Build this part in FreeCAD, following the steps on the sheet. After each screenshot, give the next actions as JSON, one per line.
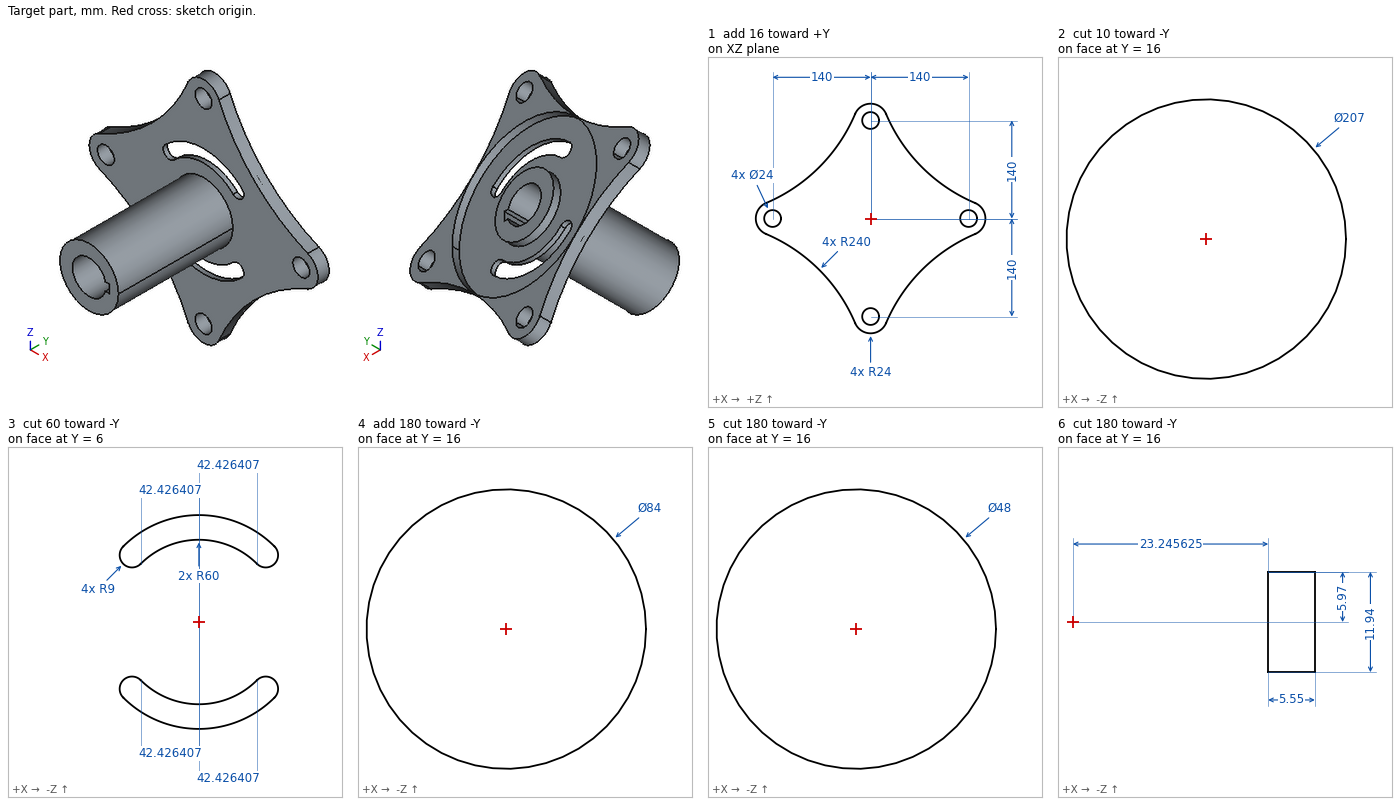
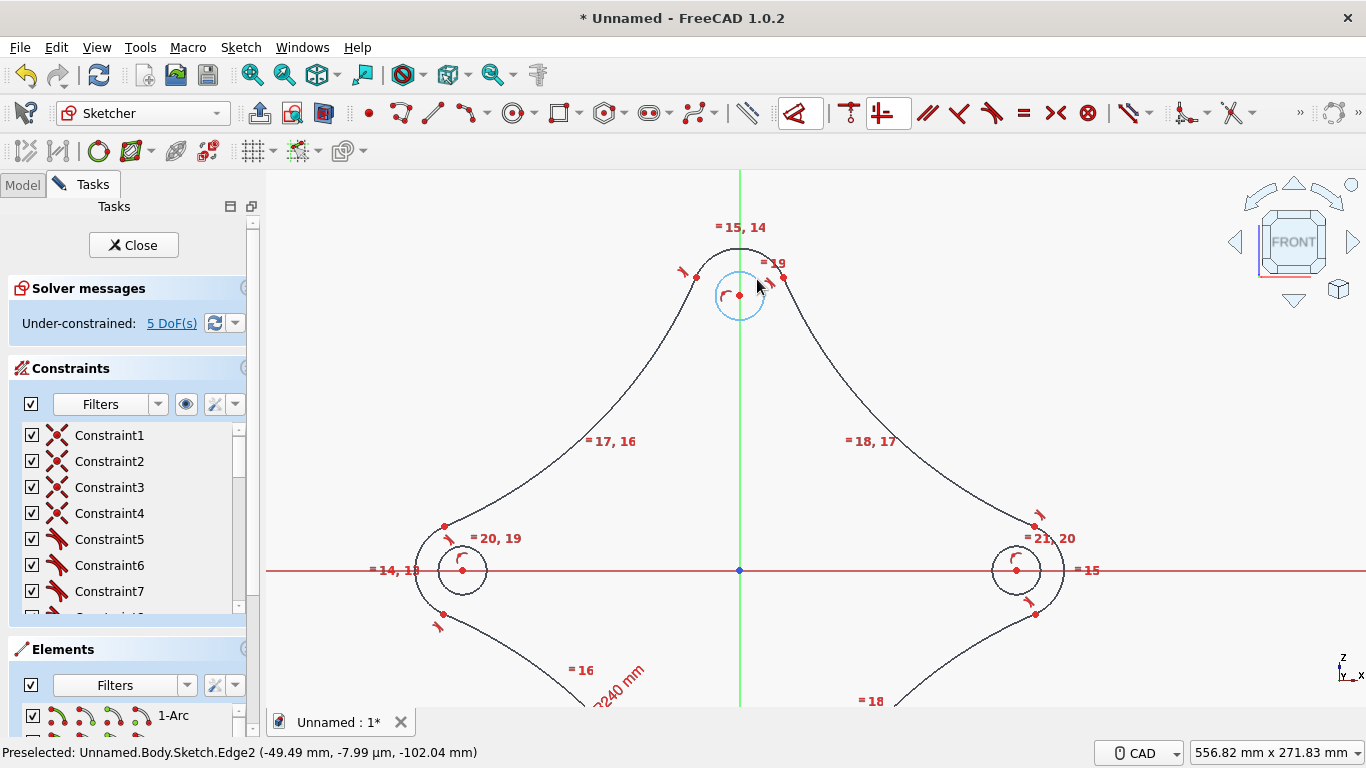
{"action": "left_click", "coordinate": [757, 279]}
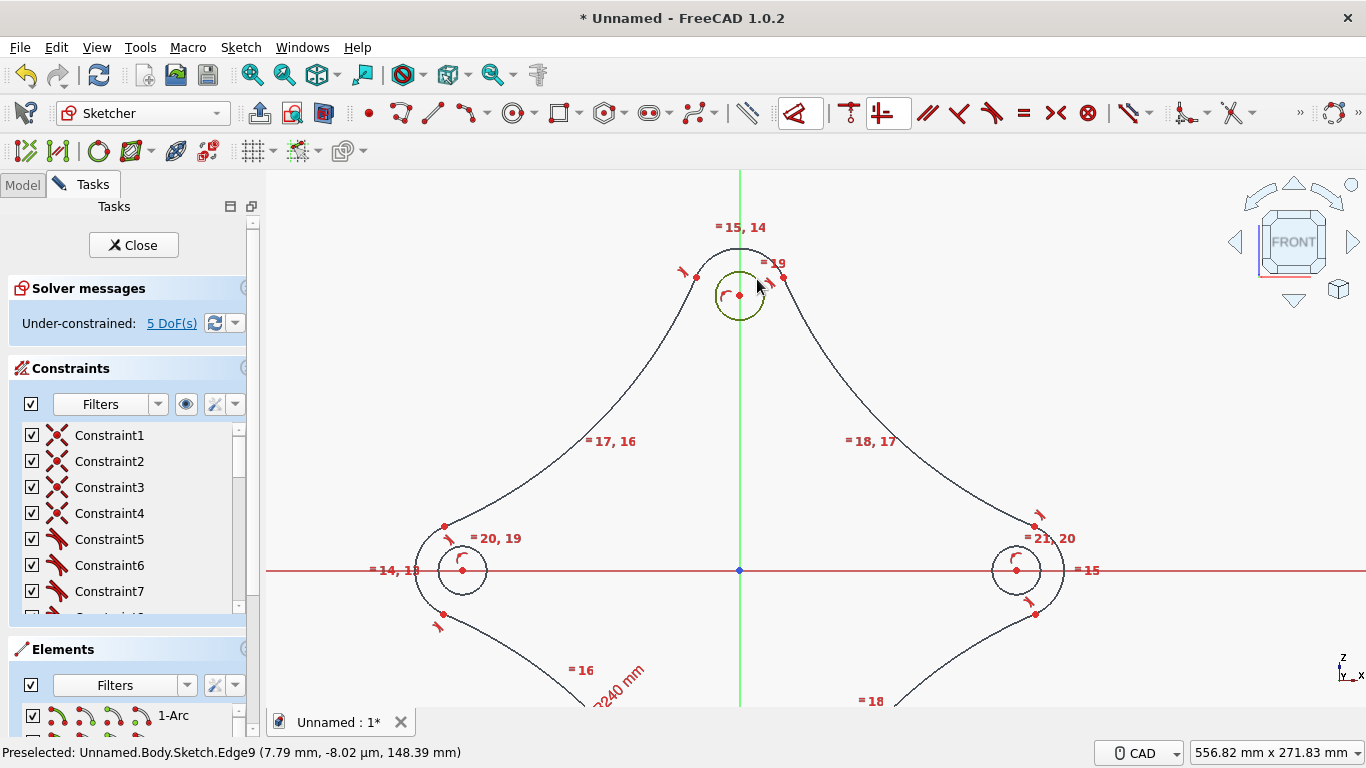
{"action": "left_click", "coordinate": [818, 114]}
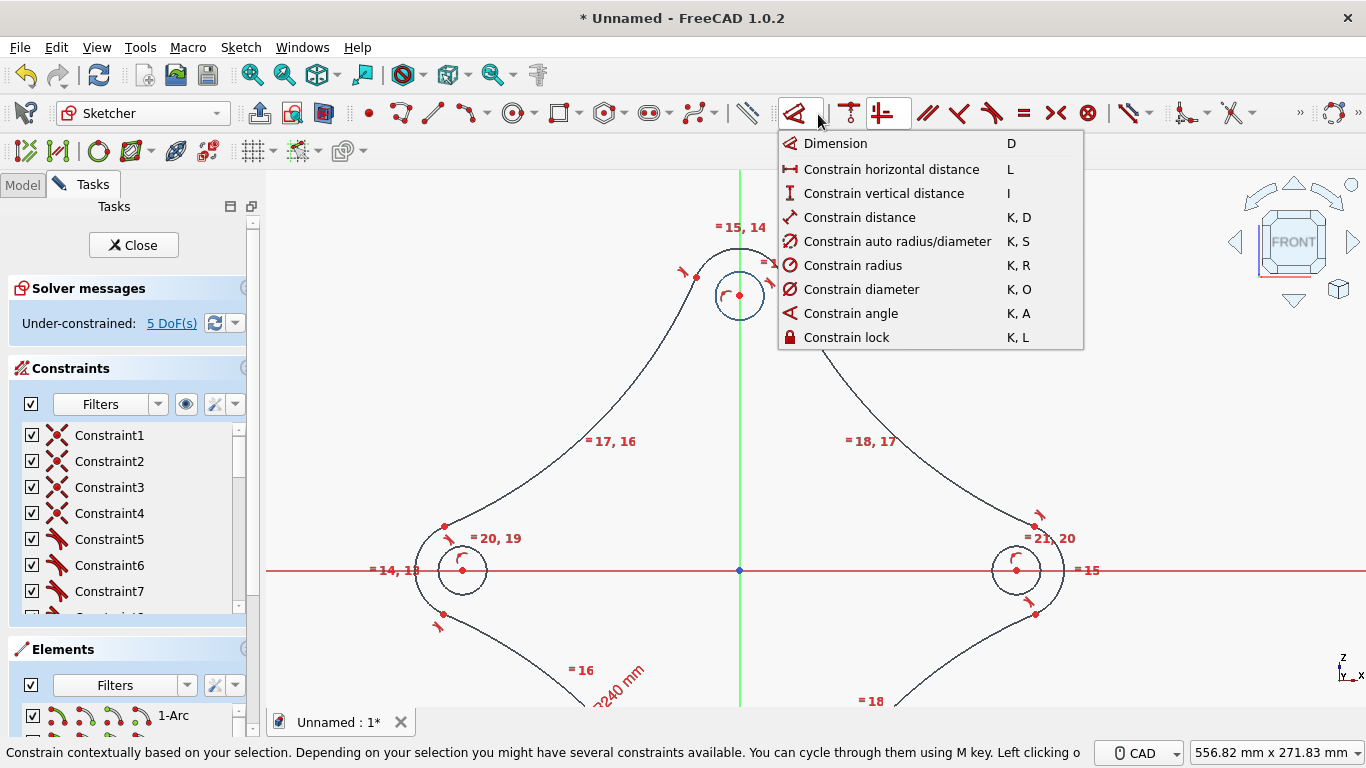
{"action": "left_click", "coordinate": [931, 289]}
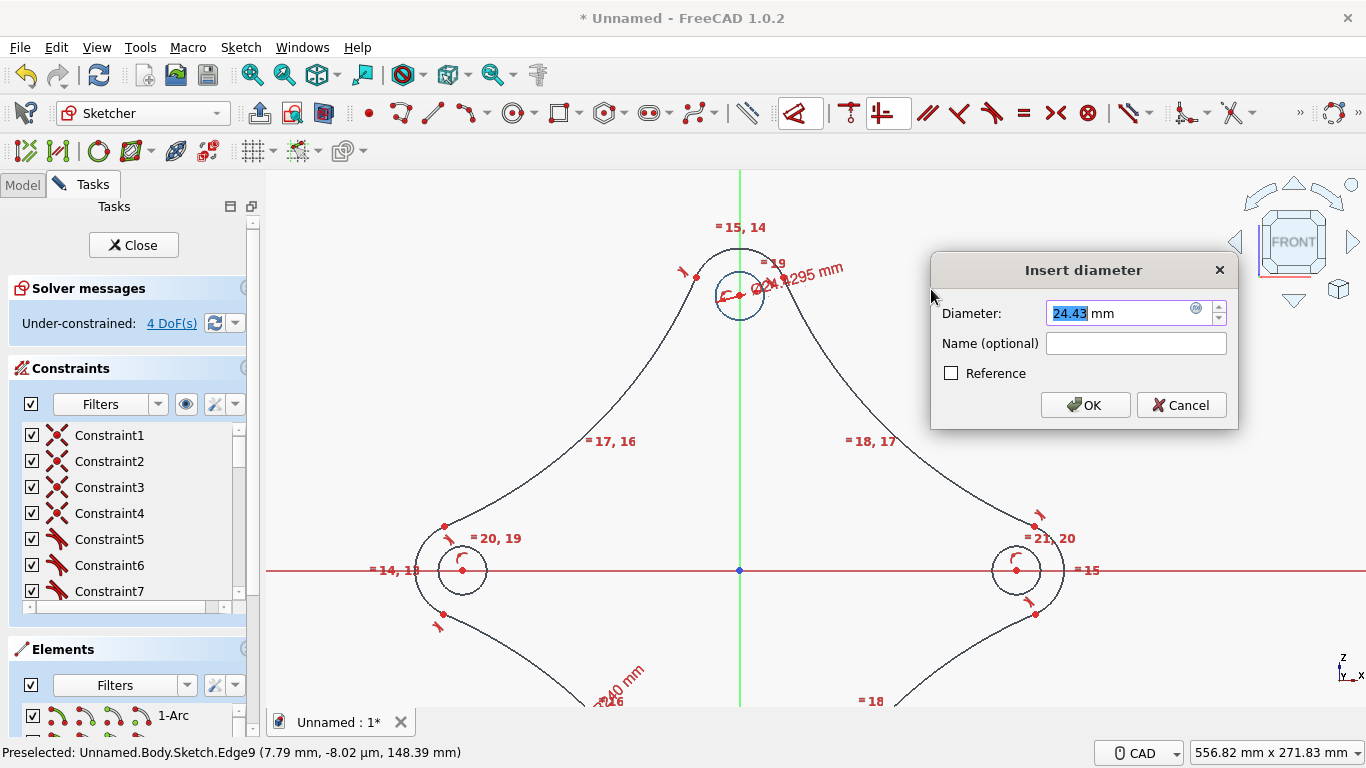
{"action": "type", "text": "24"}
{"action": "key", "text": "Return"}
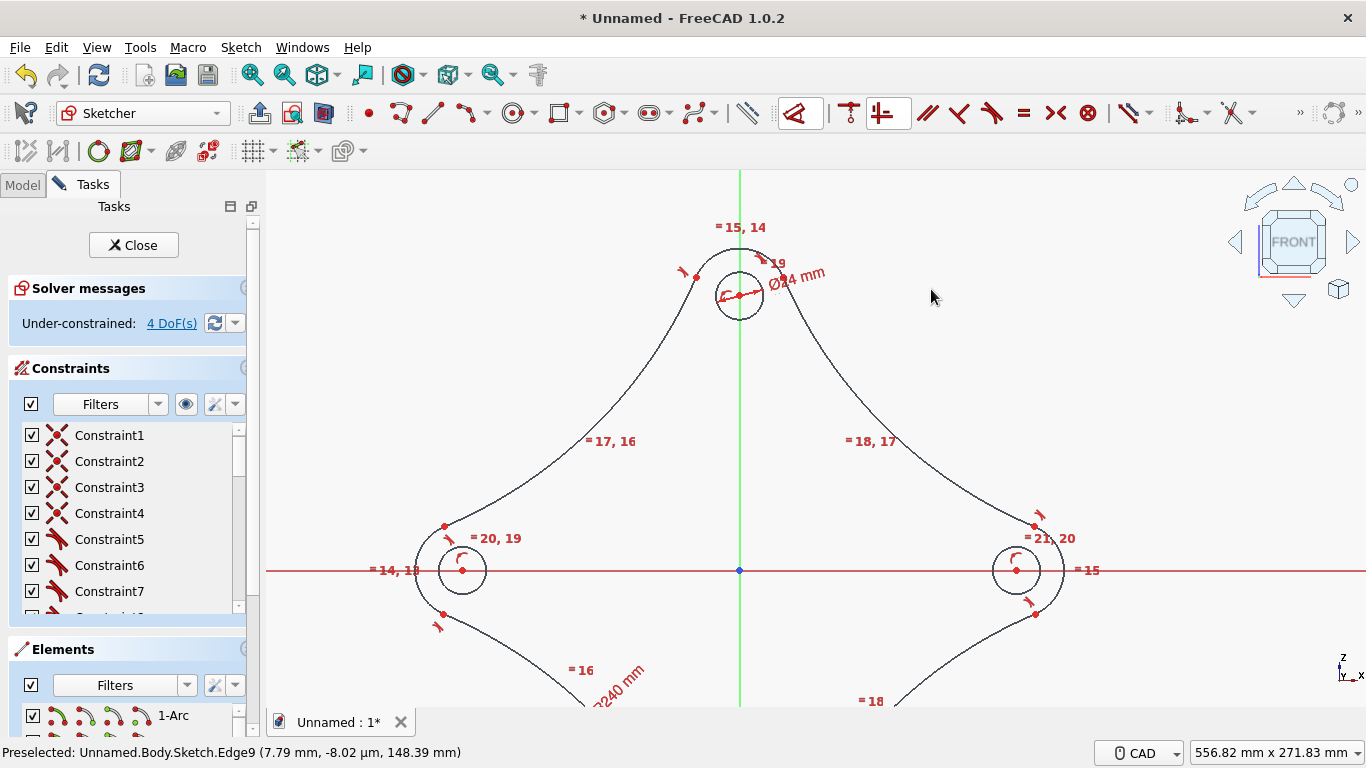
{"action": "left_click", "coordinate": [740, 296]}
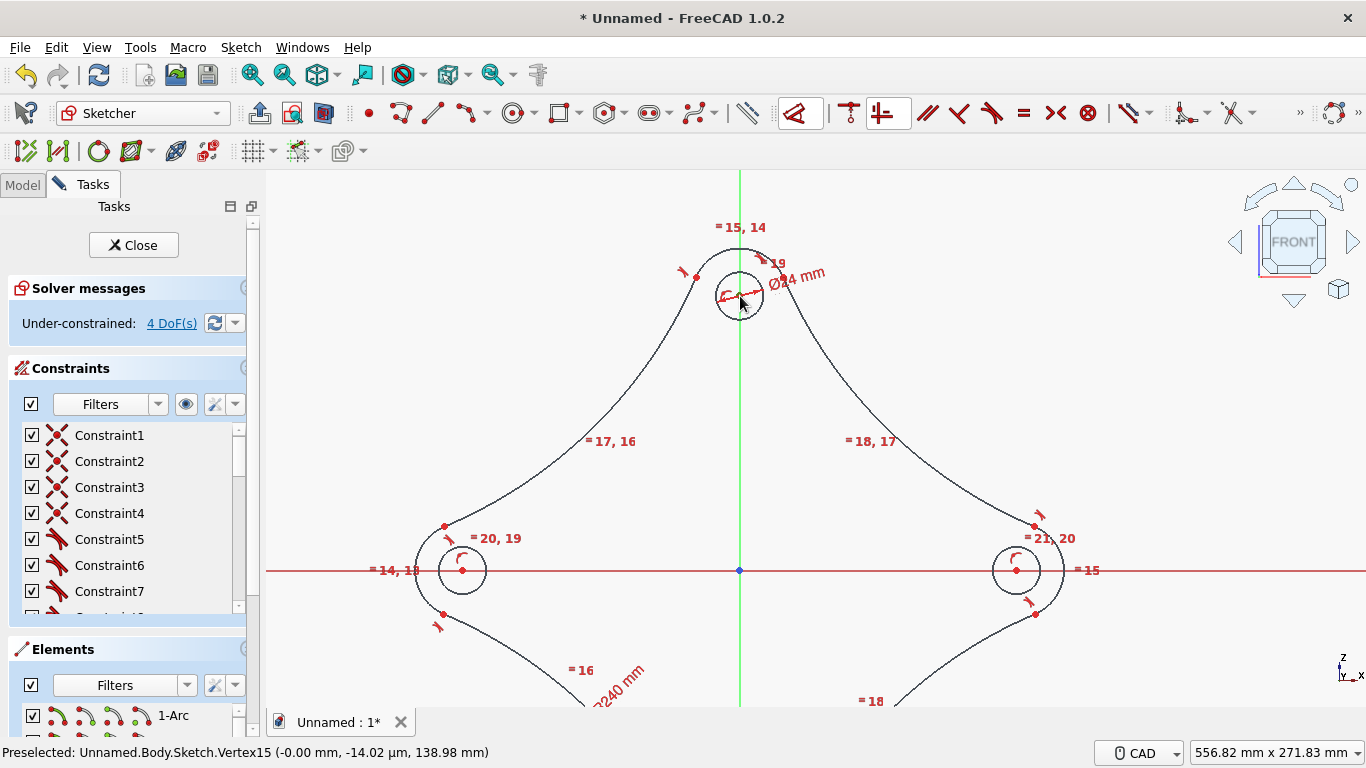
{"action": "key", "text": "i"}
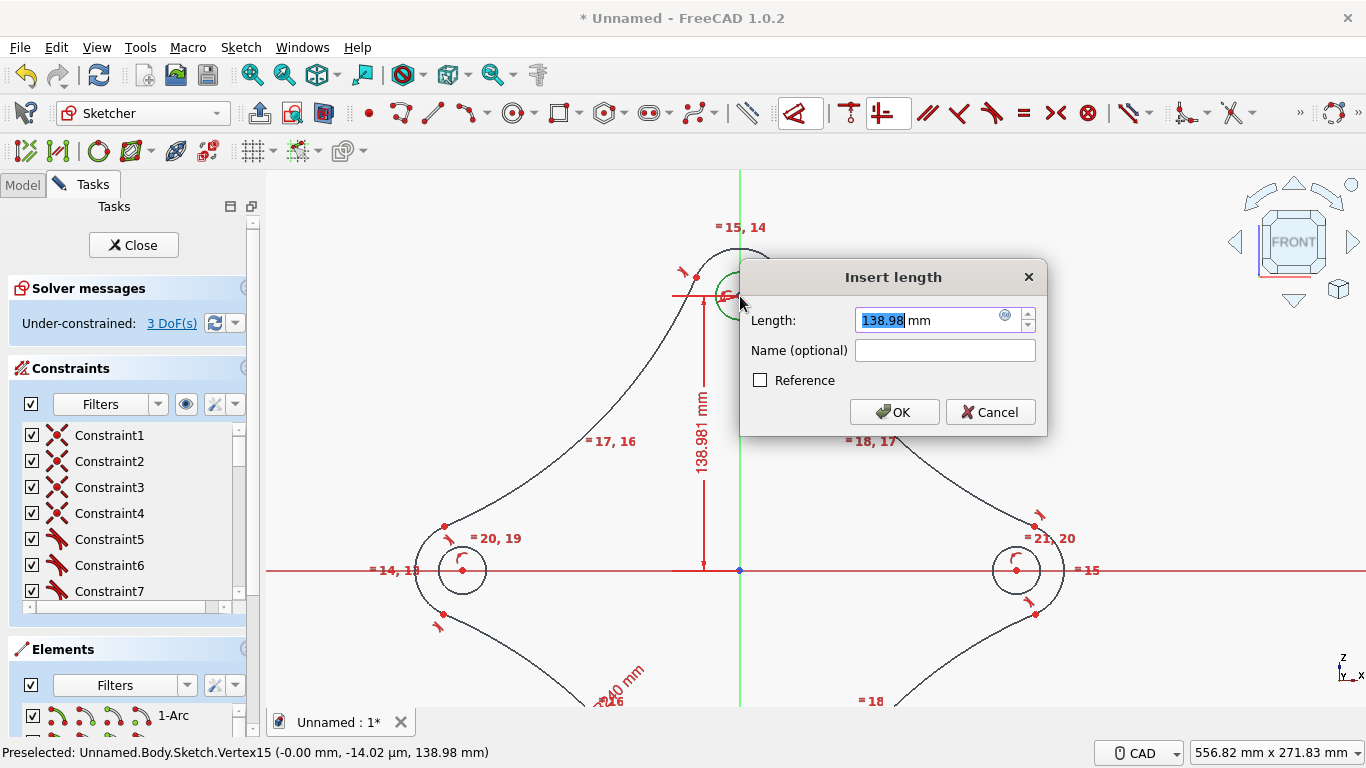
{"action": "type", "text": "140"}
{"action": "key", "text": "Return"}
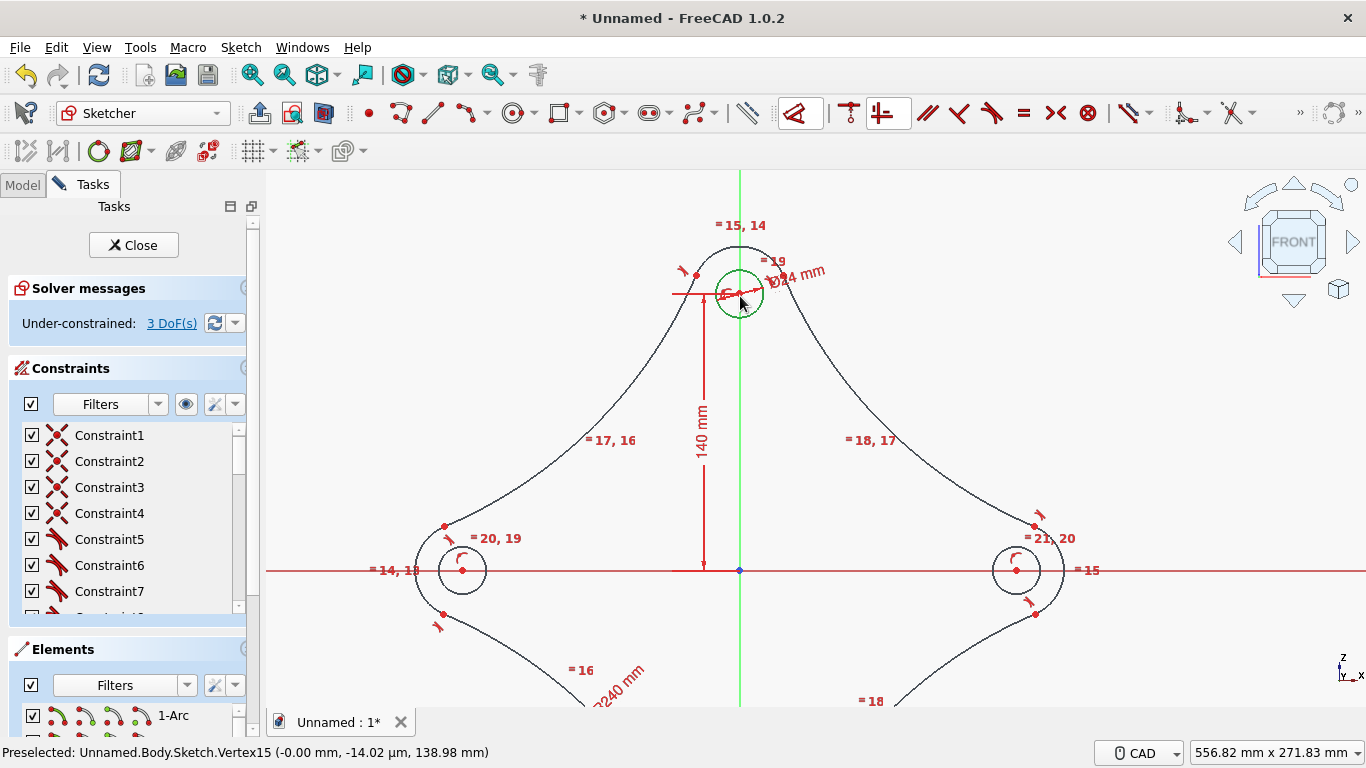
{"action": "left_click", "coordinate": [463, 571]}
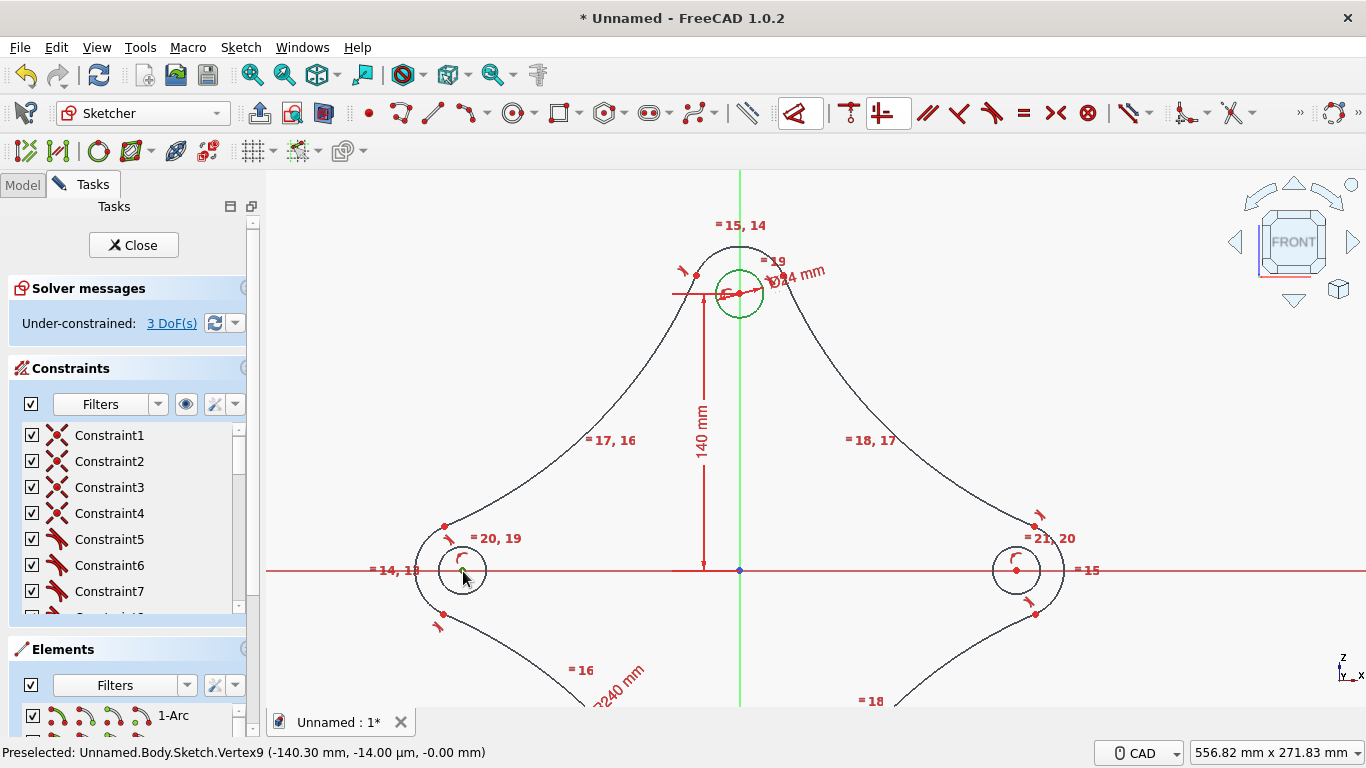
{"action": "left_click", "coordinate": [818, 114]}